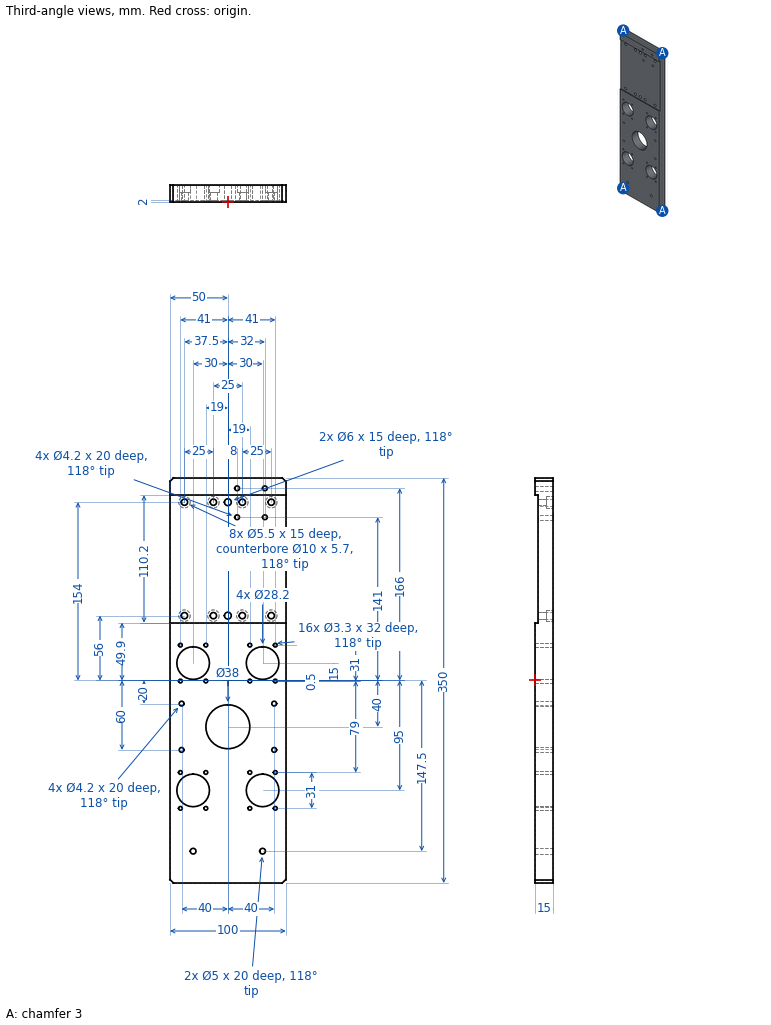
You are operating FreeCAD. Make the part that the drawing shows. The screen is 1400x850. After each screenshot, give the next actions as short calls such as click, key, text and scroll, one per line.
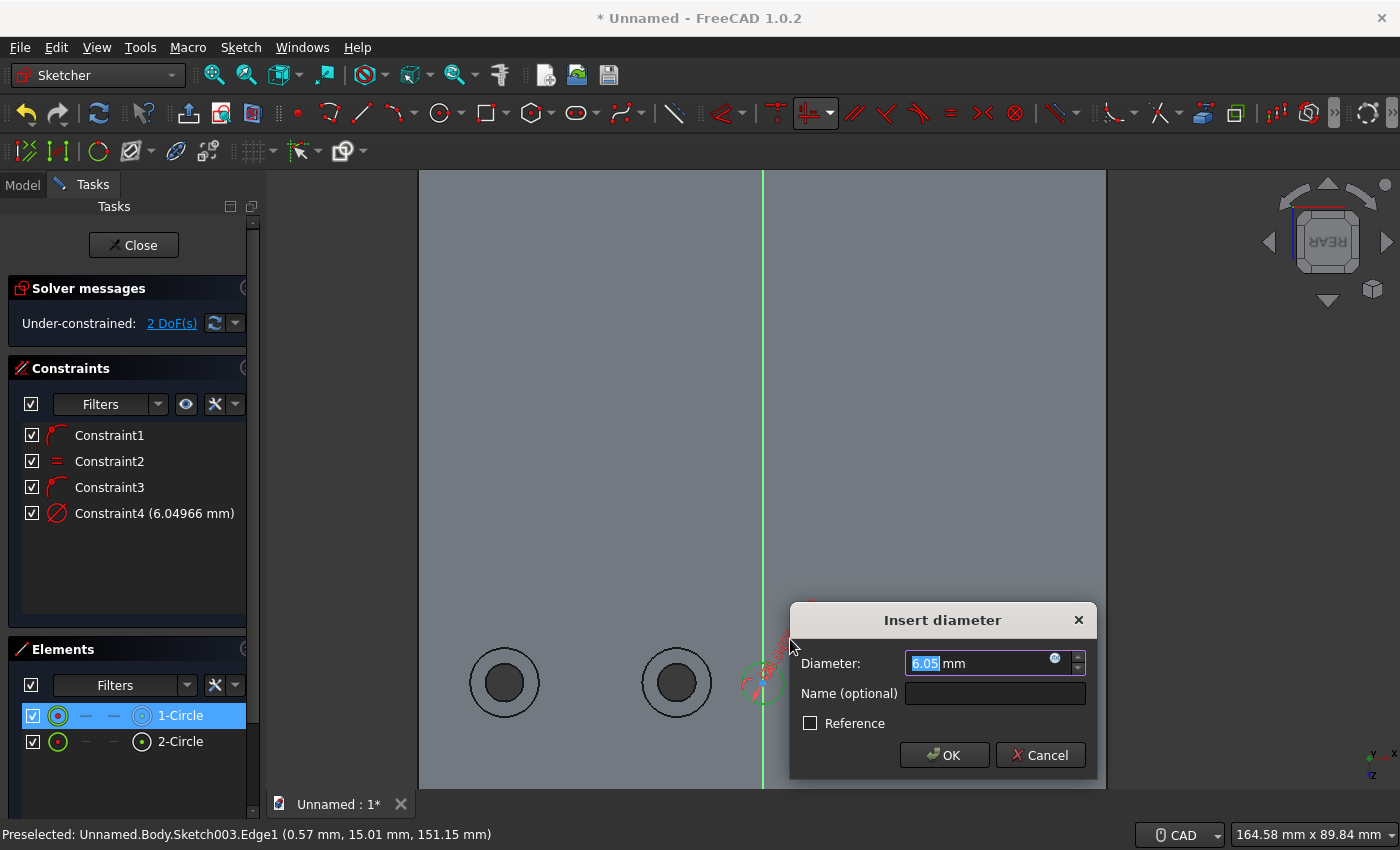
text(6)
key(Return)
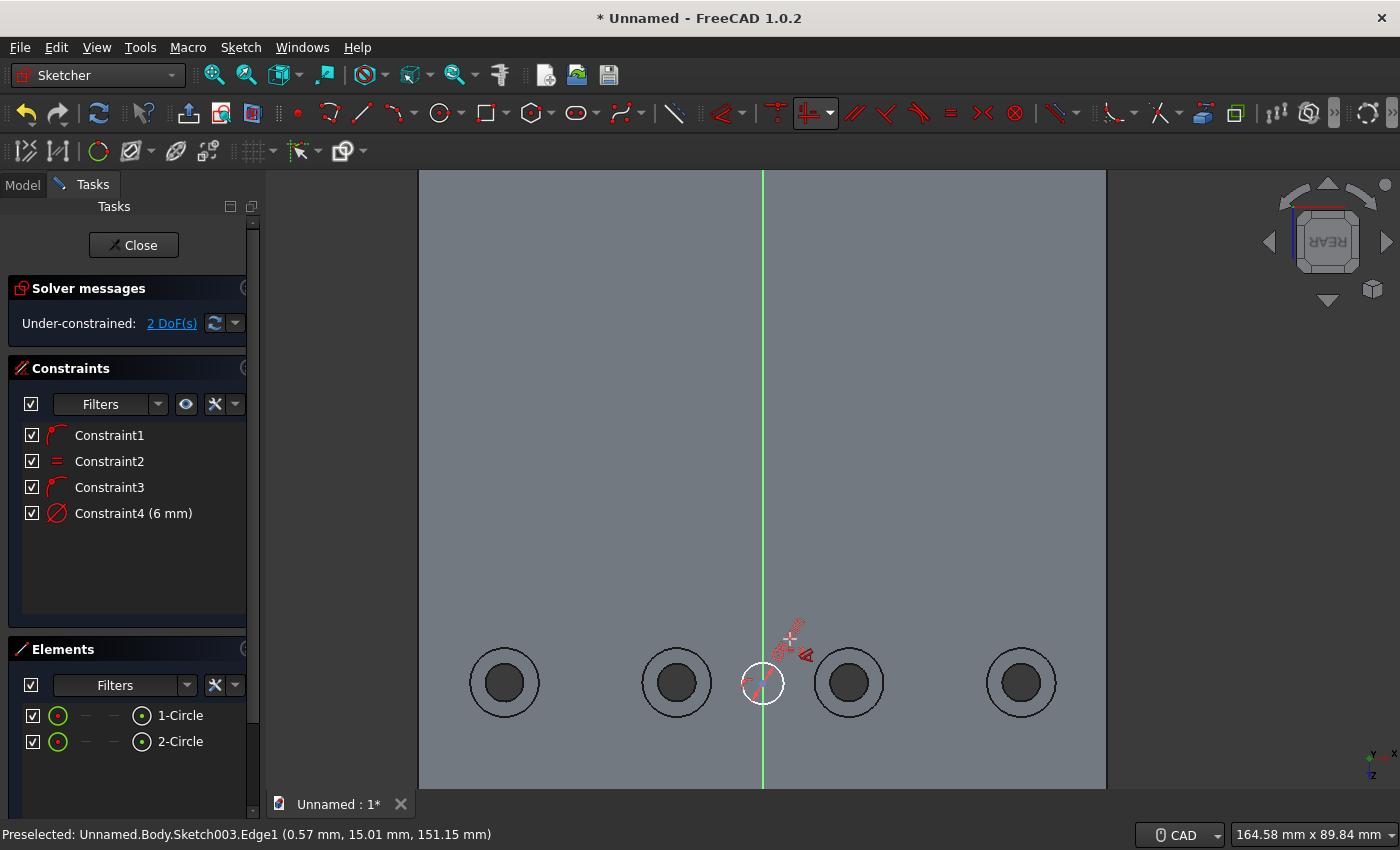
scroll(765, 664, down, 5)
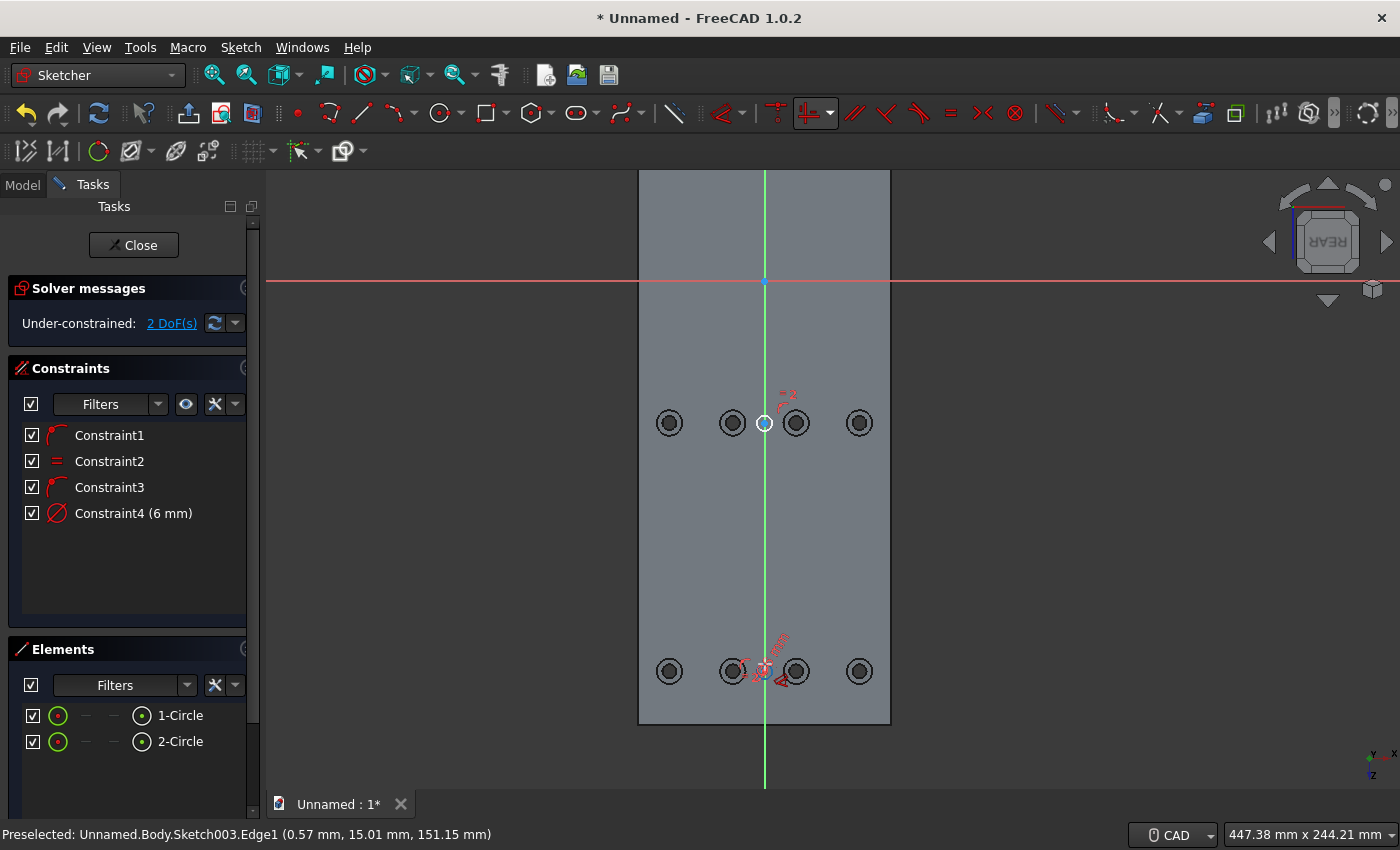
click(765, 423)
click(799, 352)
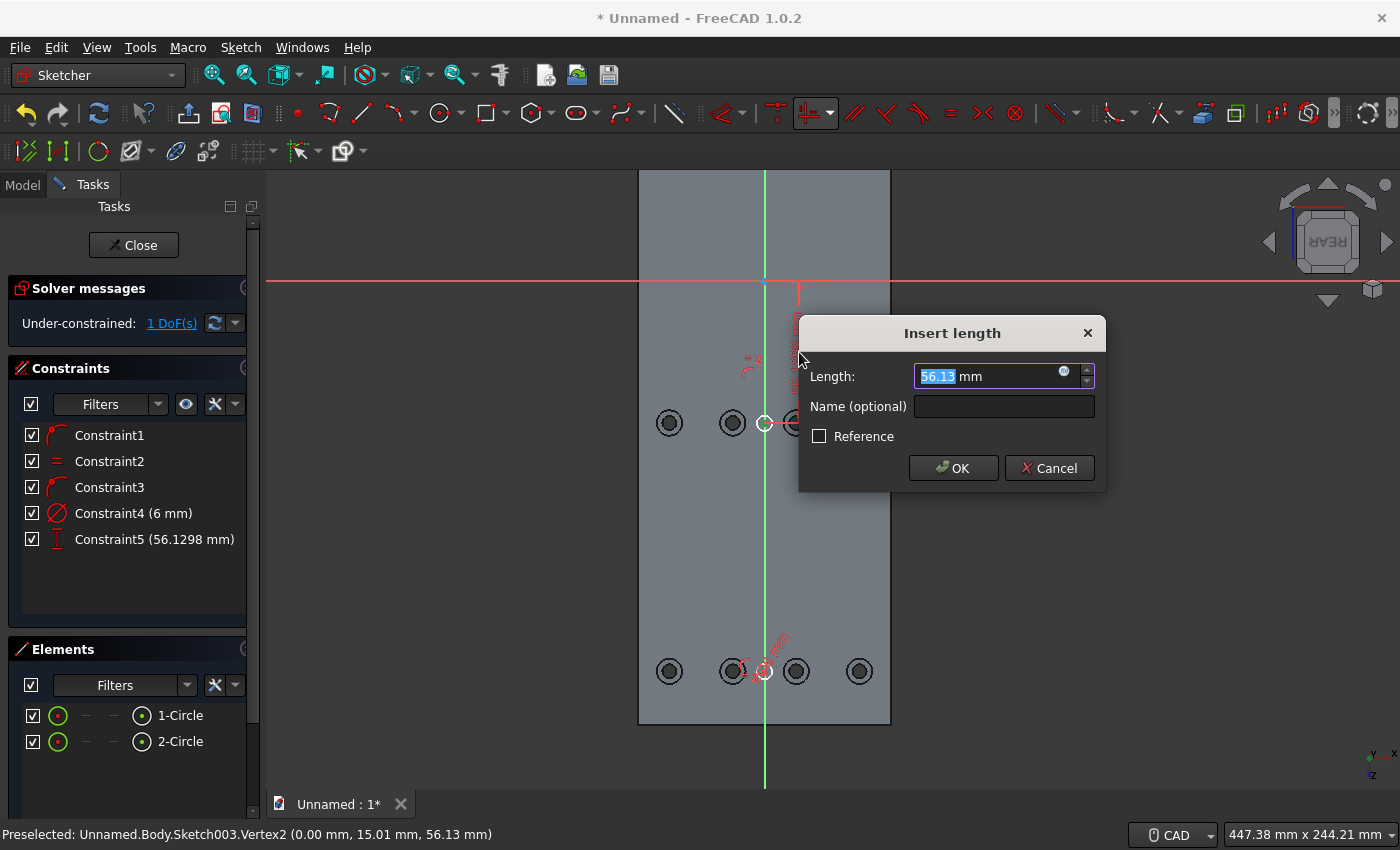
text(56)
key(Return)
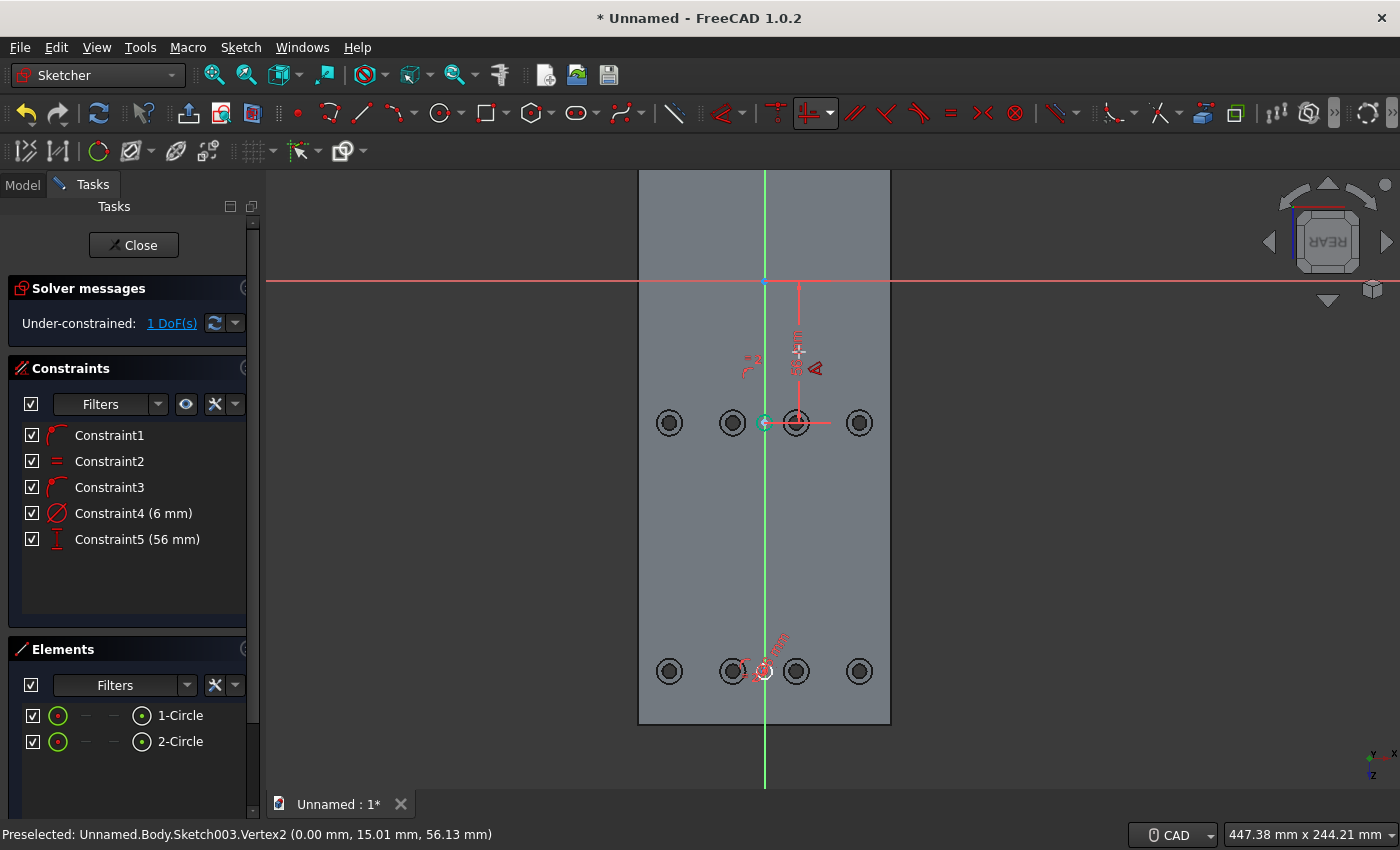
click(765, 672)
click(799, 476)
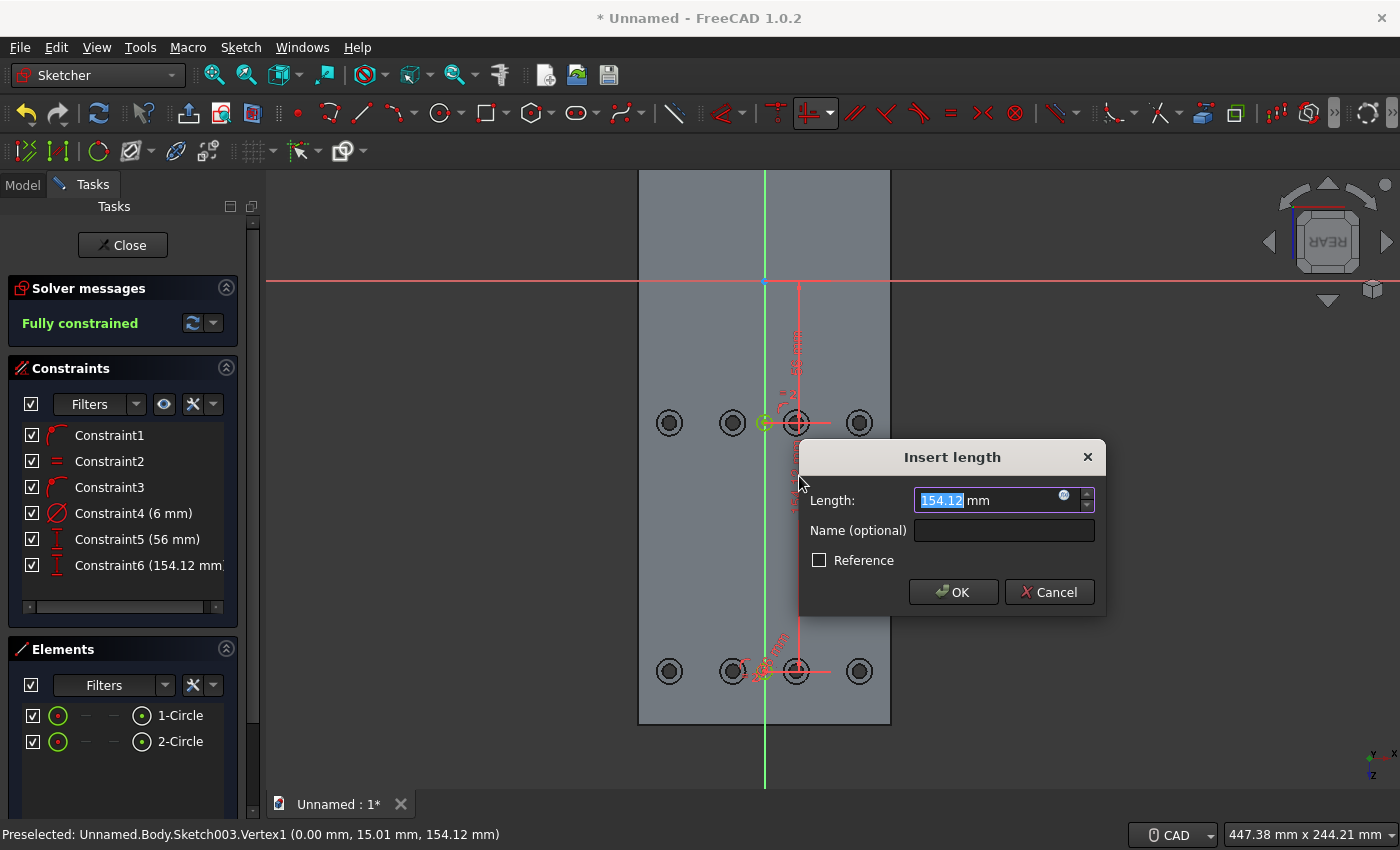
text(154)
key(Return)
key(Escape)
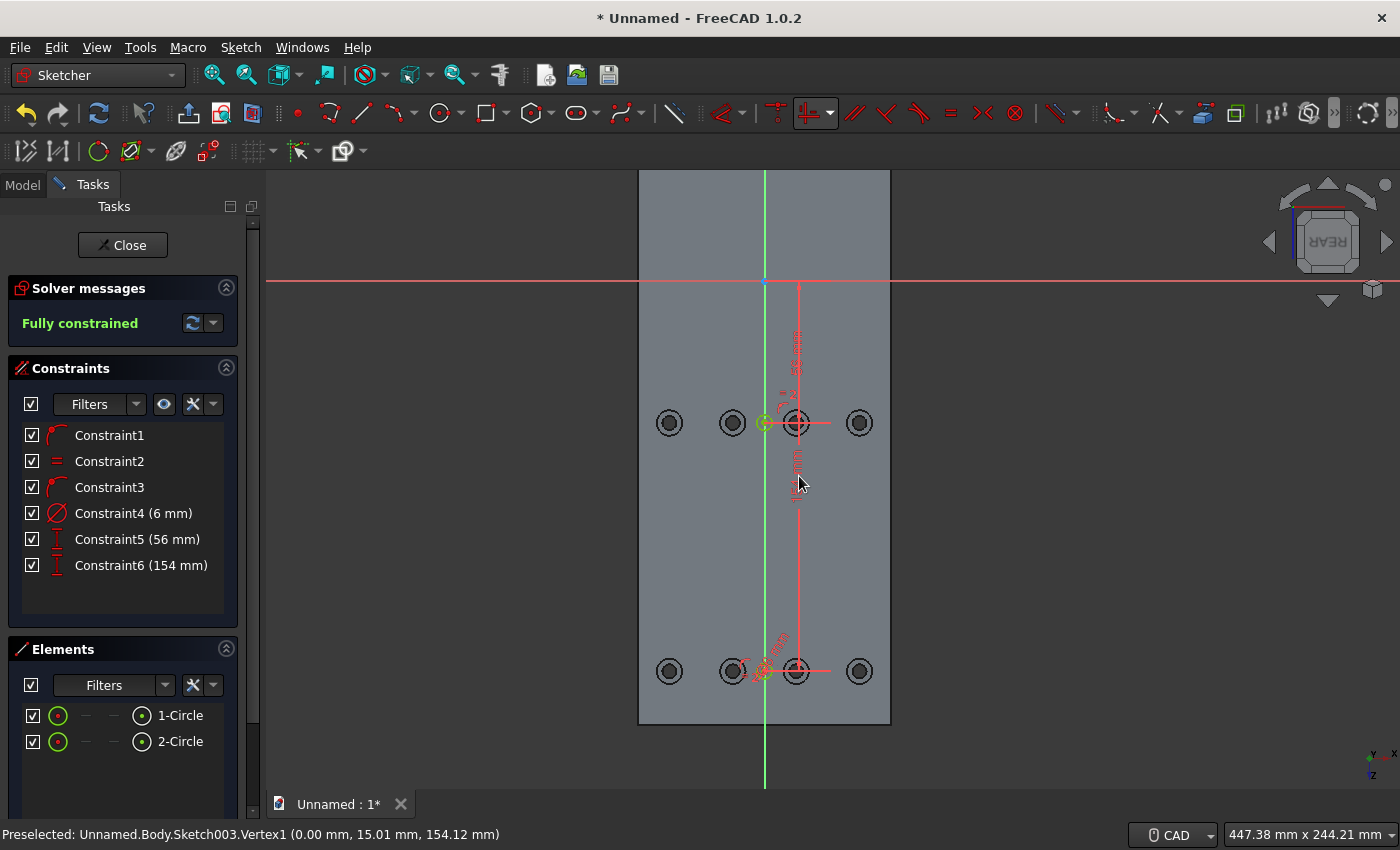
click(123, 245)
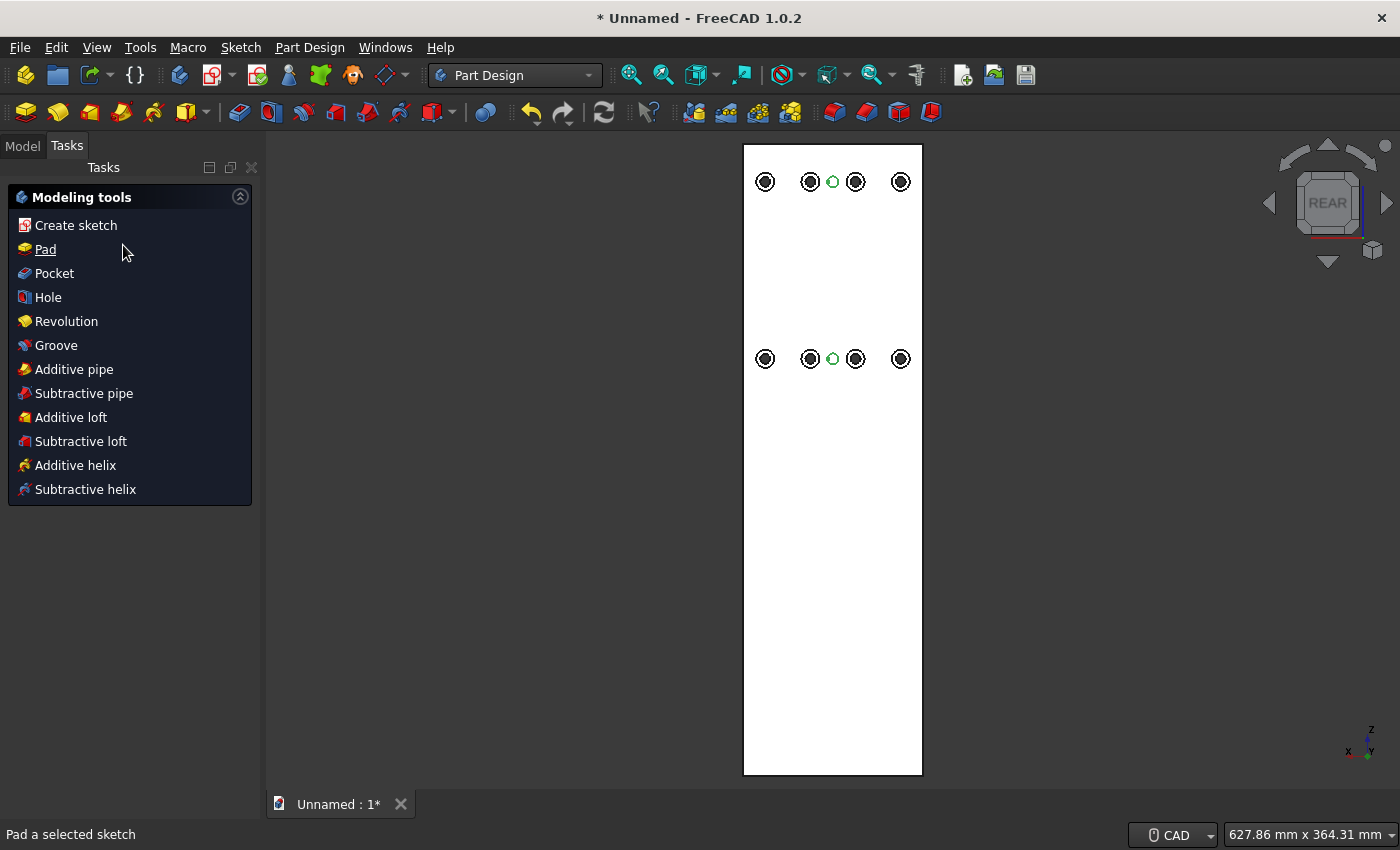
click(272, 112)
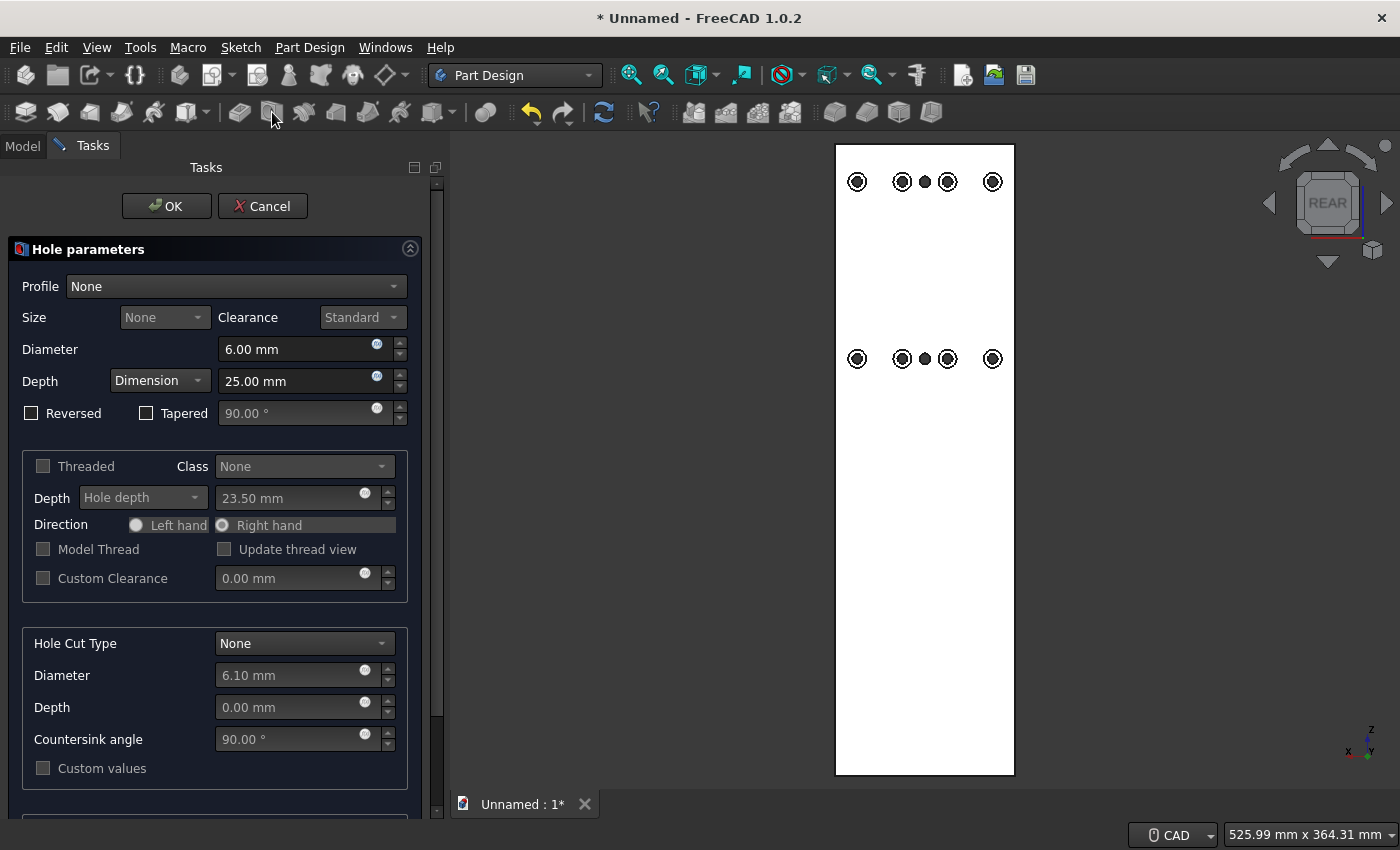
triple_click(305, 349)